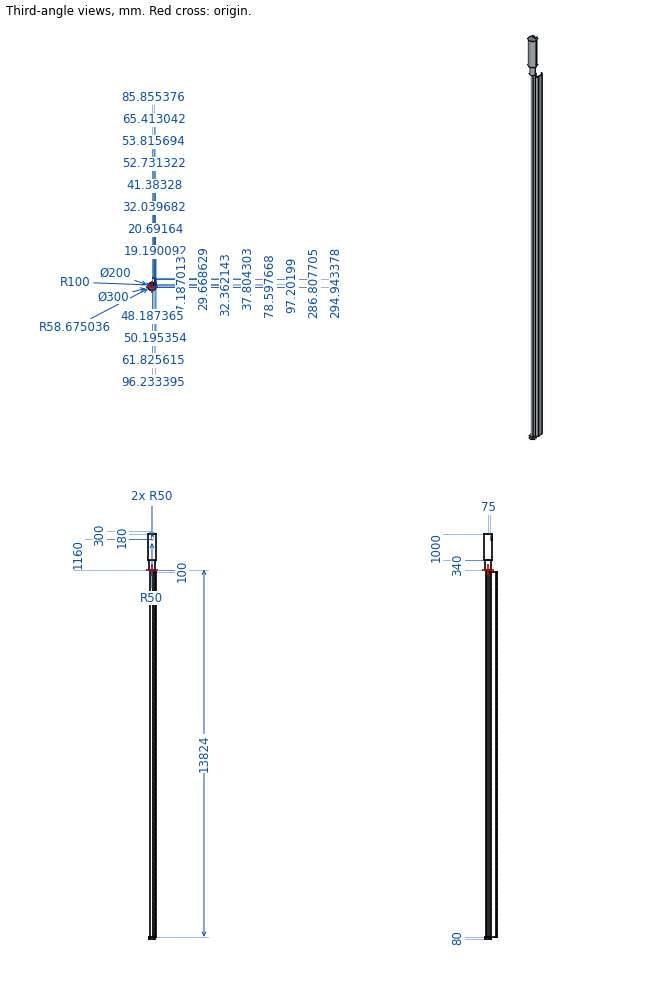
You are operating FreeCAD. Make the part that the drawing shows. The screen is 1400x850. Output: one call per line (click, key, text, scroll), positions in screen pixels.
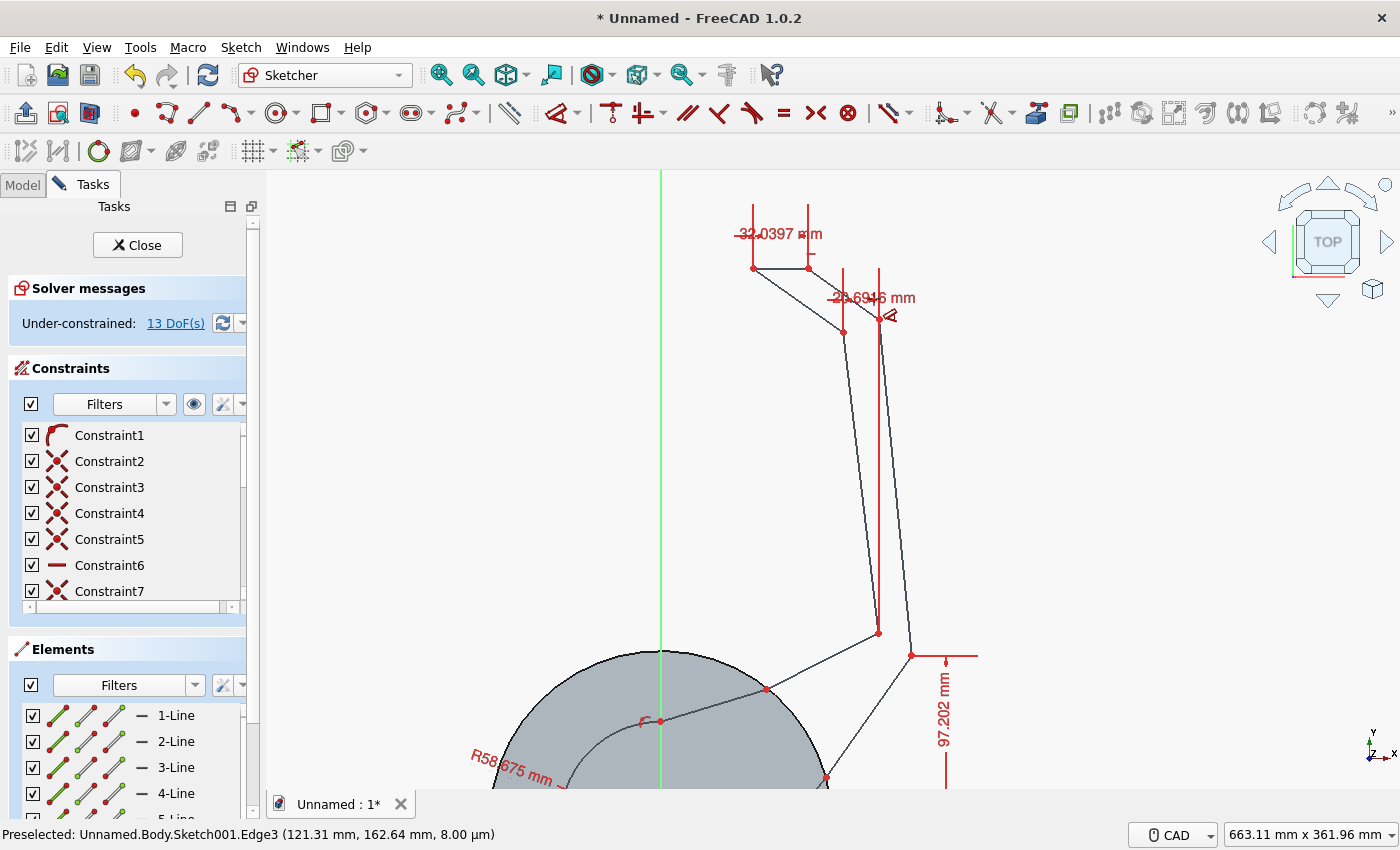
click(829, 284)
click(860, 235)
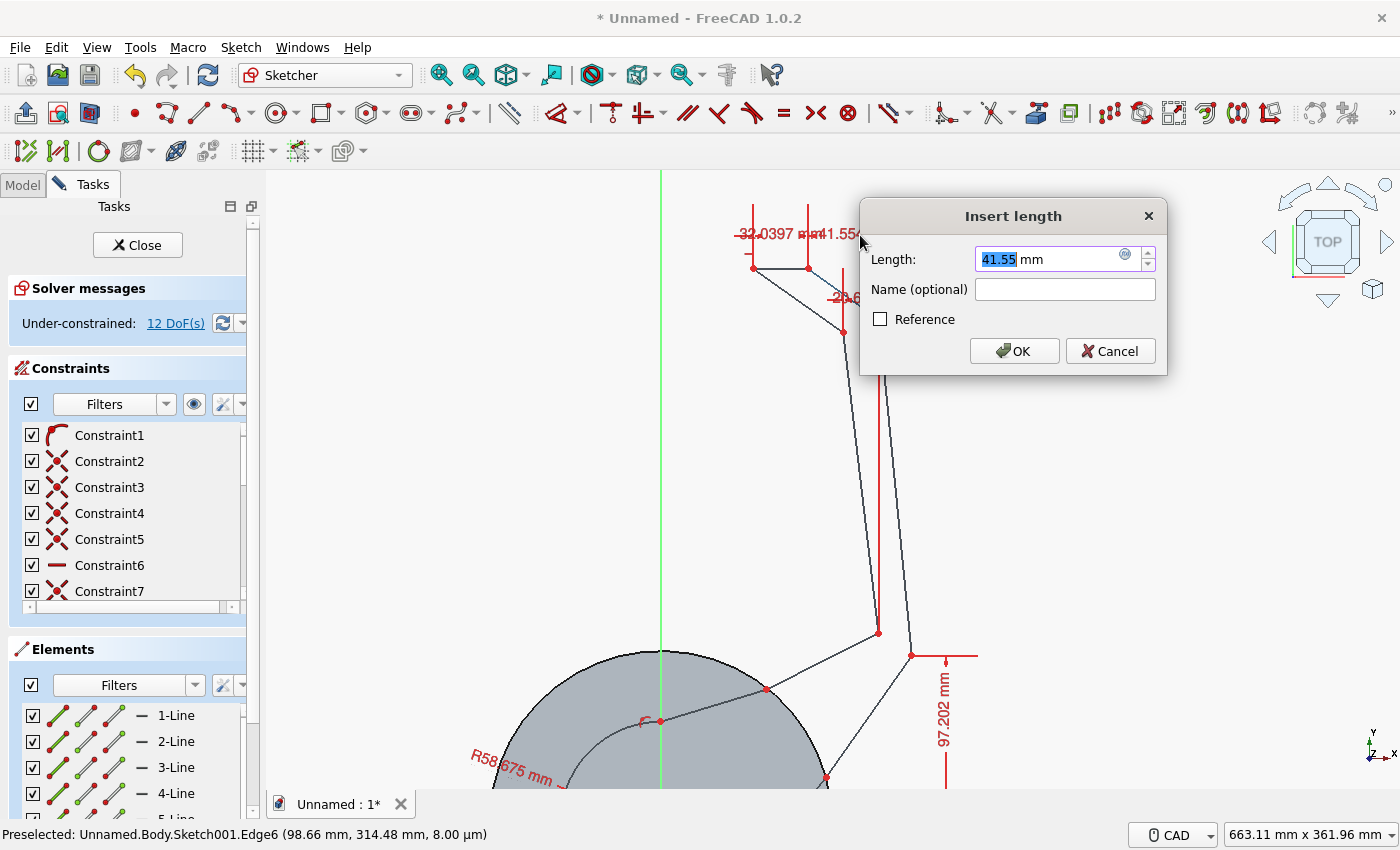
text(41.38328)
key(Return)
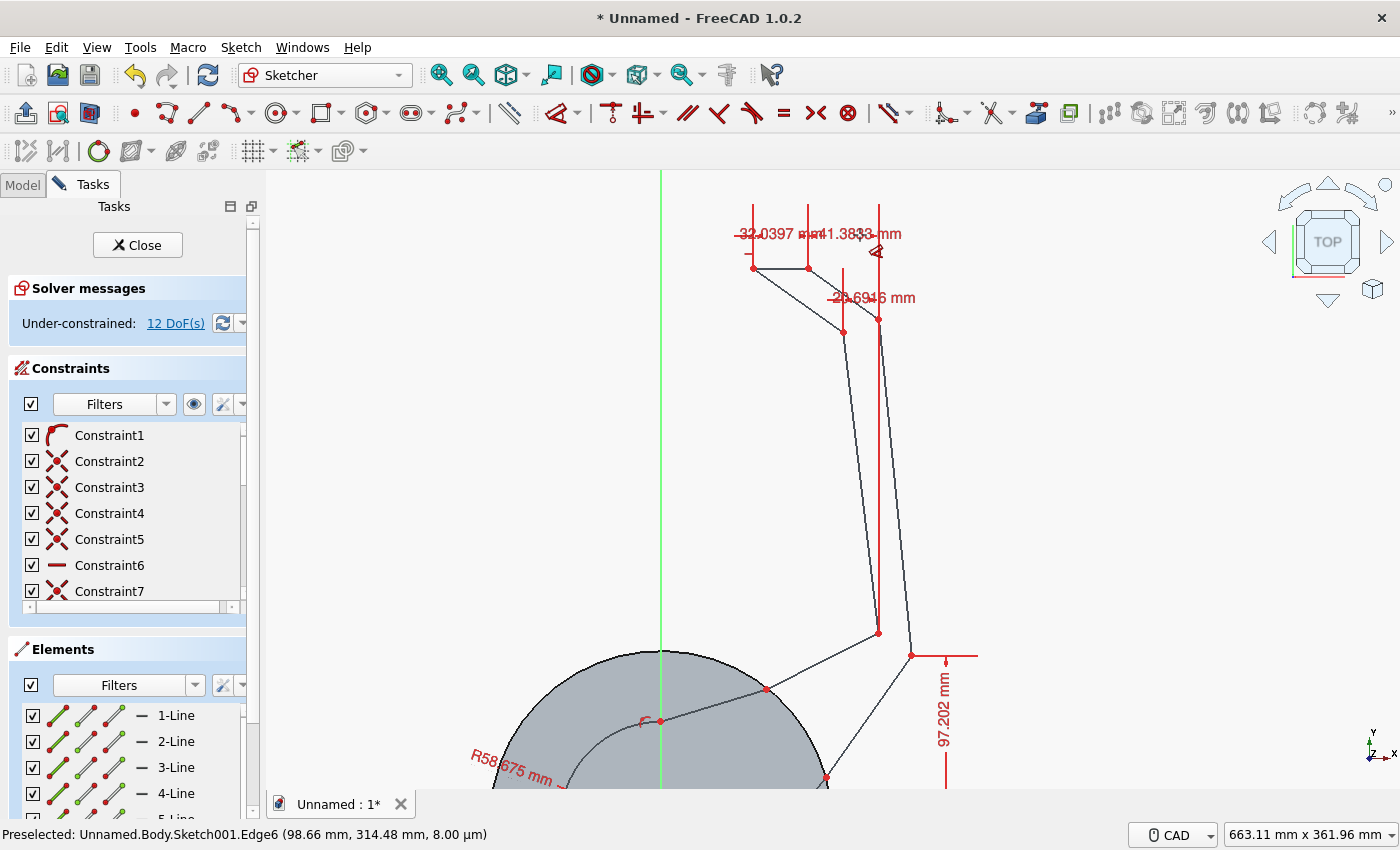
click(766, 690)
click(713, 656)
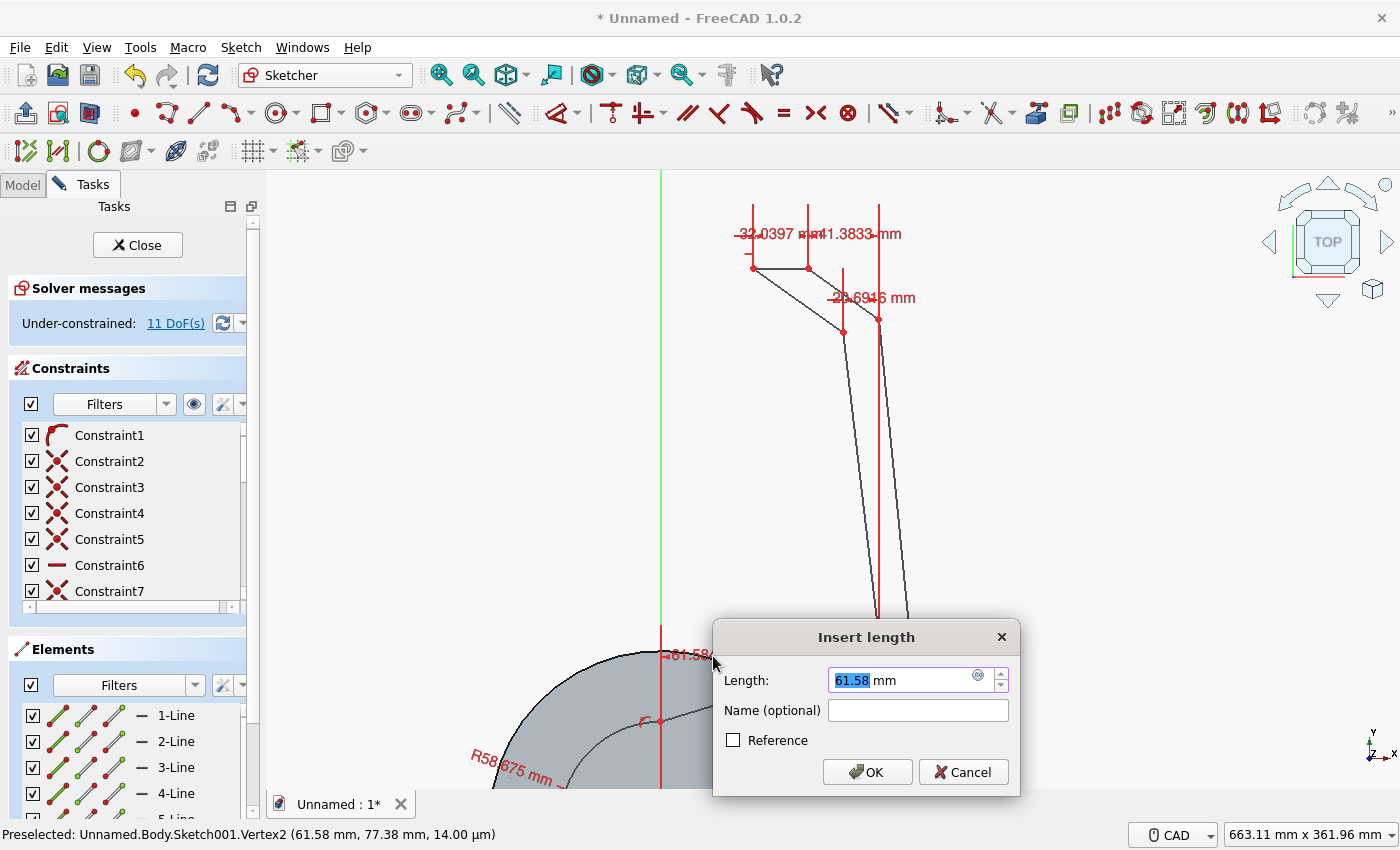
text(61.825615)
key(Return)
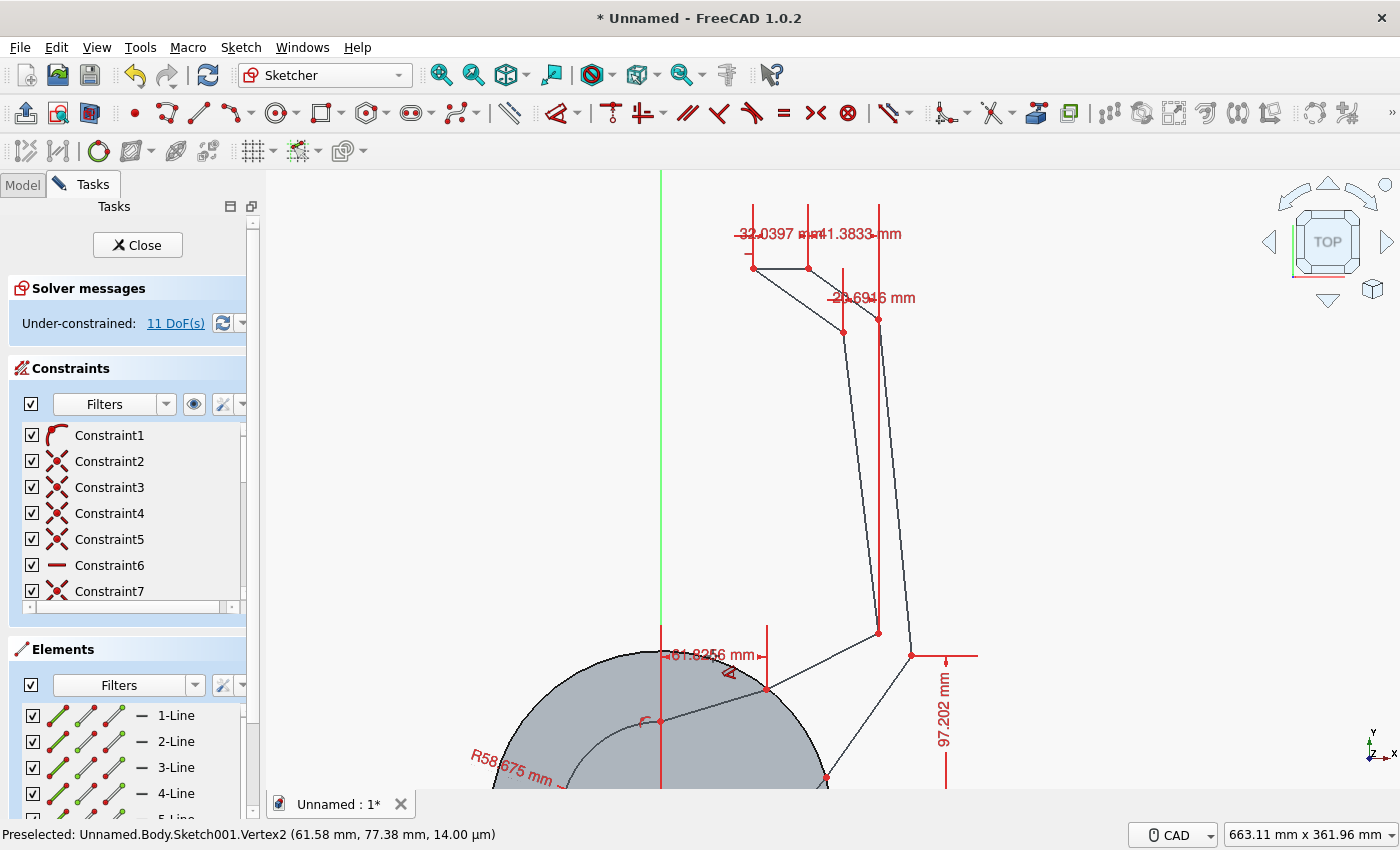
click(767, 690)
click(627, 709)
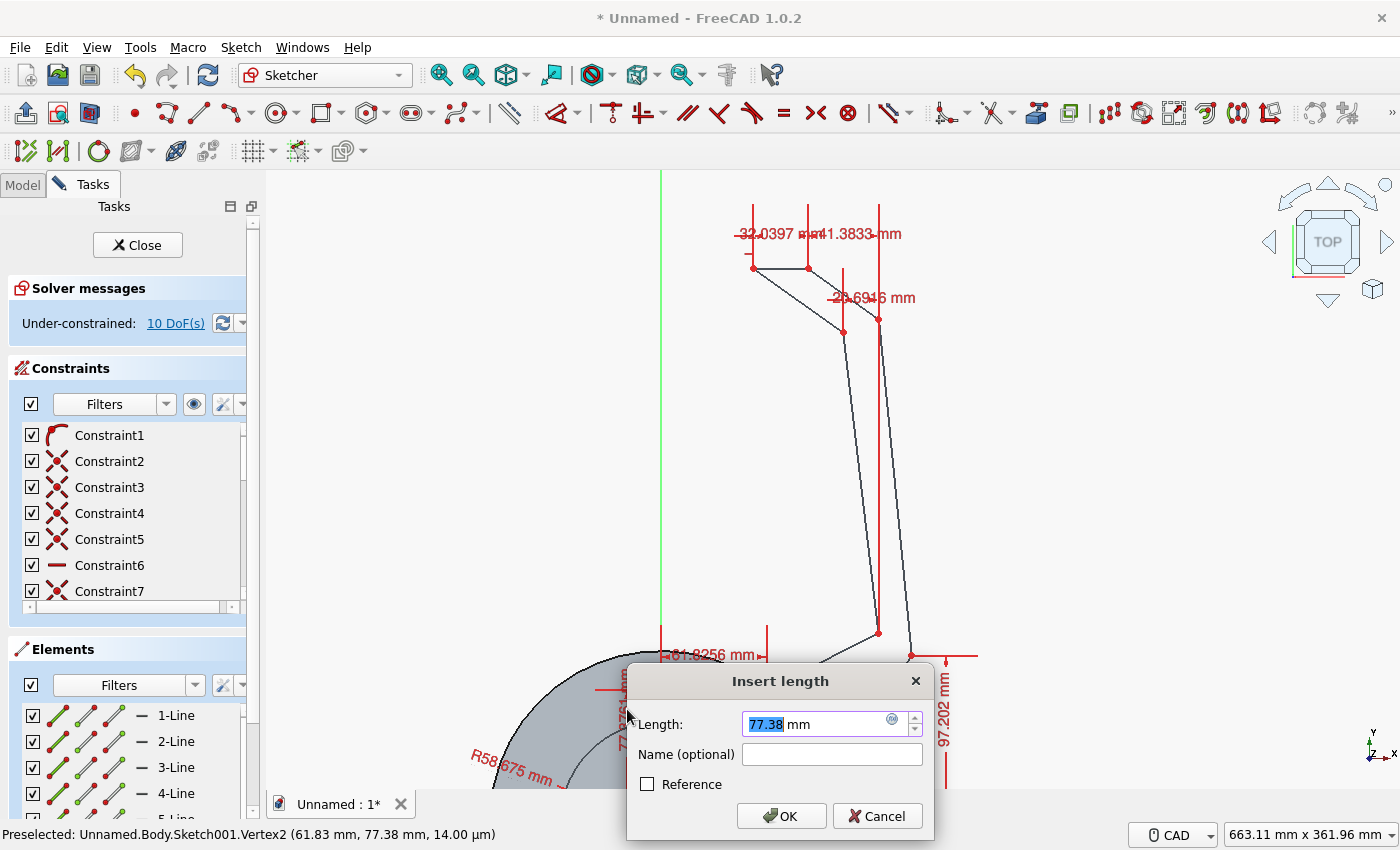
text(78.597668)
key(Return)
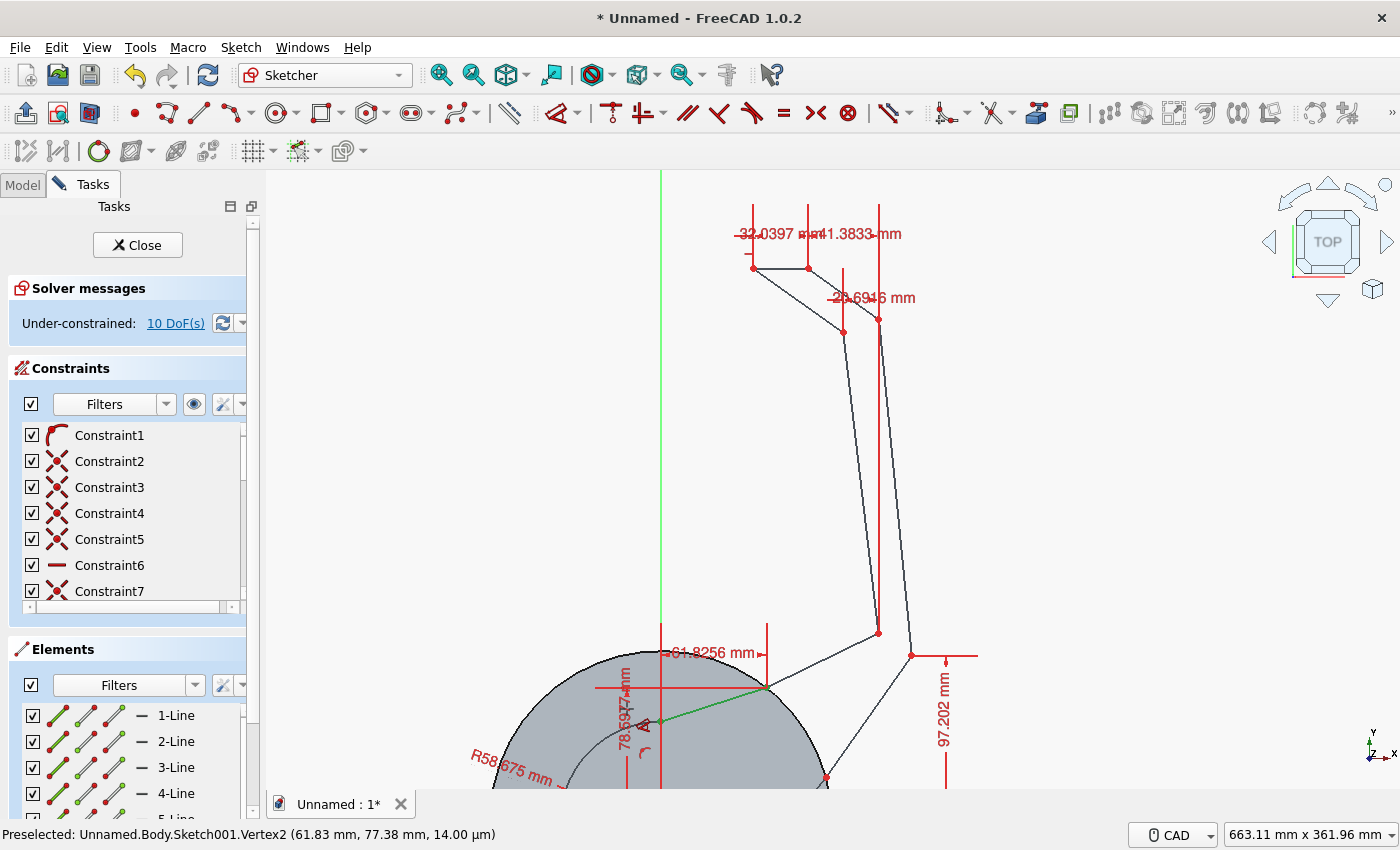
click(753, 269)
click(707, 235)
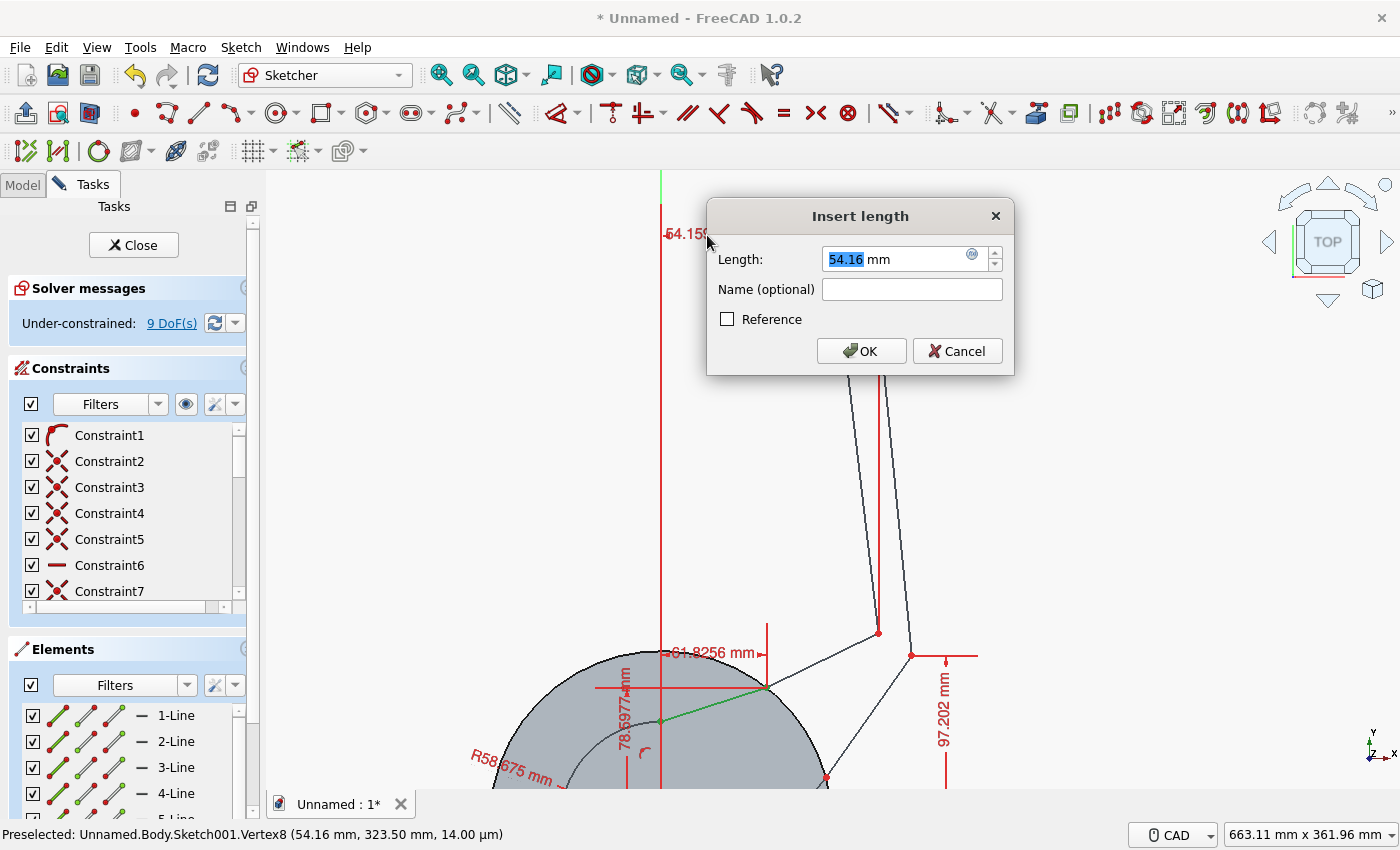
text(53.815694)
key(Return)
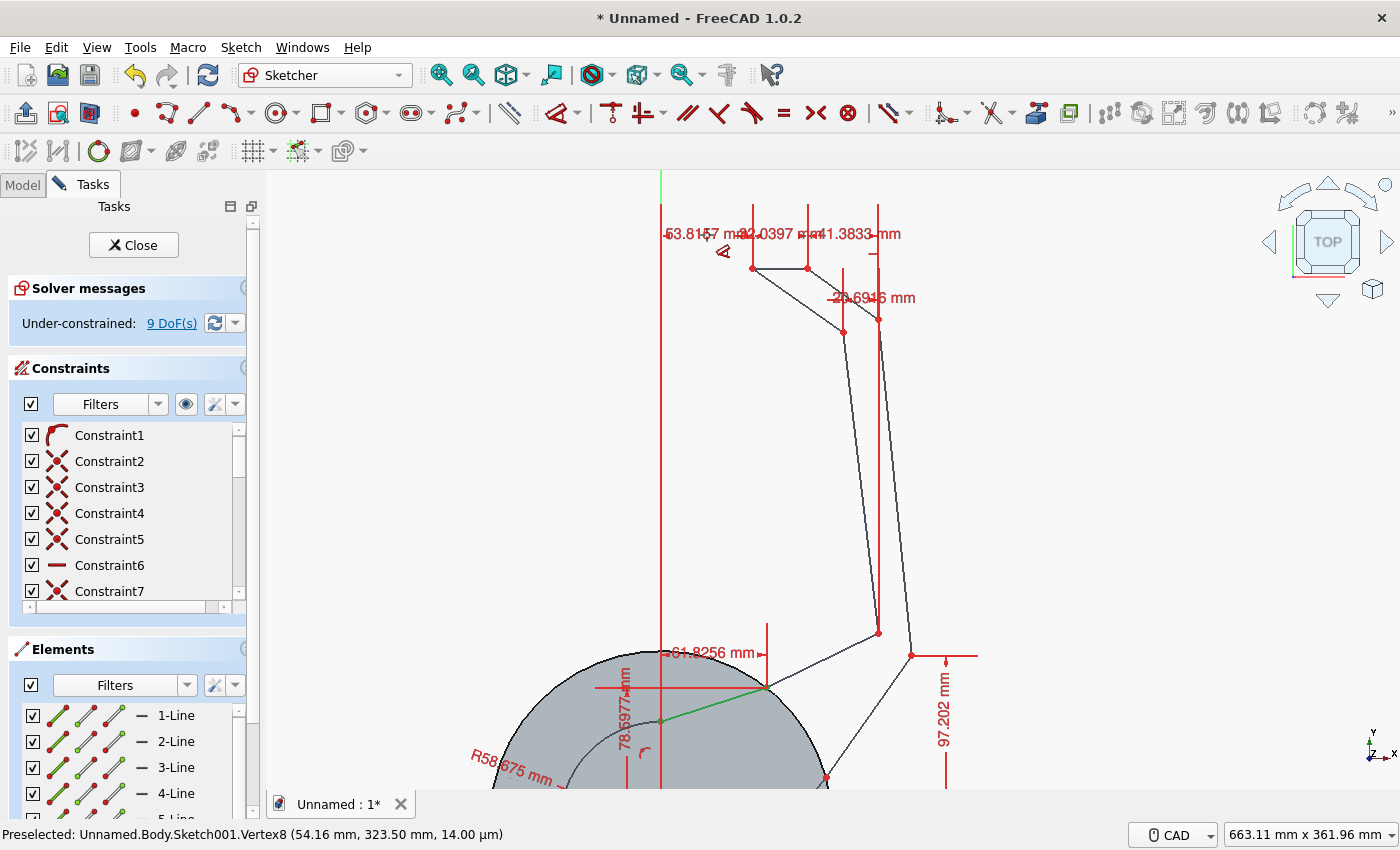
scroll(811, 289, down, 2)